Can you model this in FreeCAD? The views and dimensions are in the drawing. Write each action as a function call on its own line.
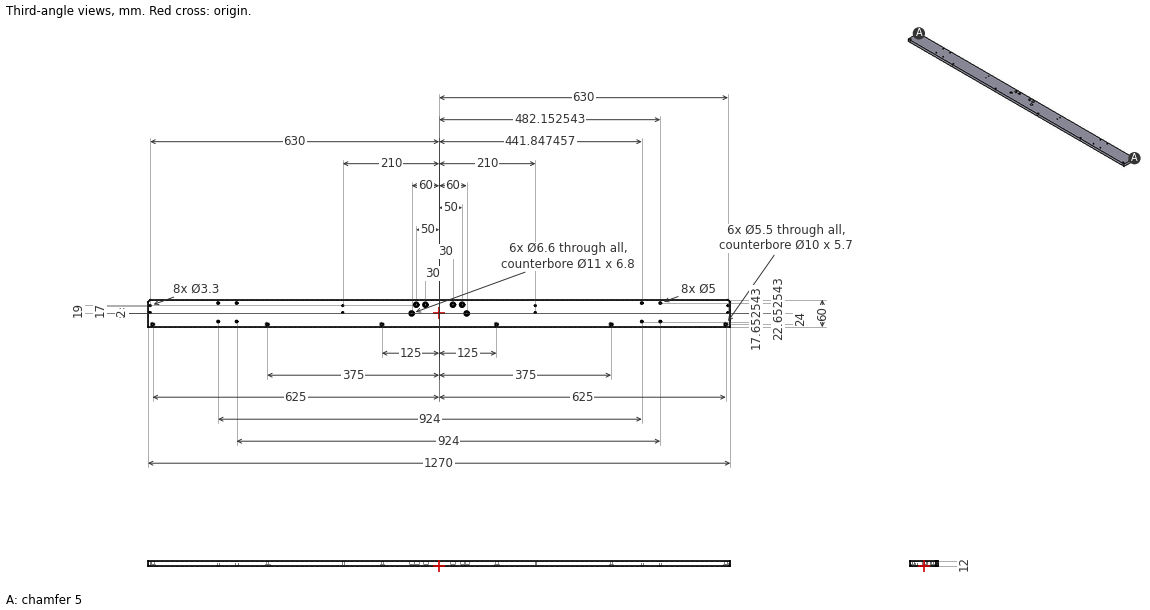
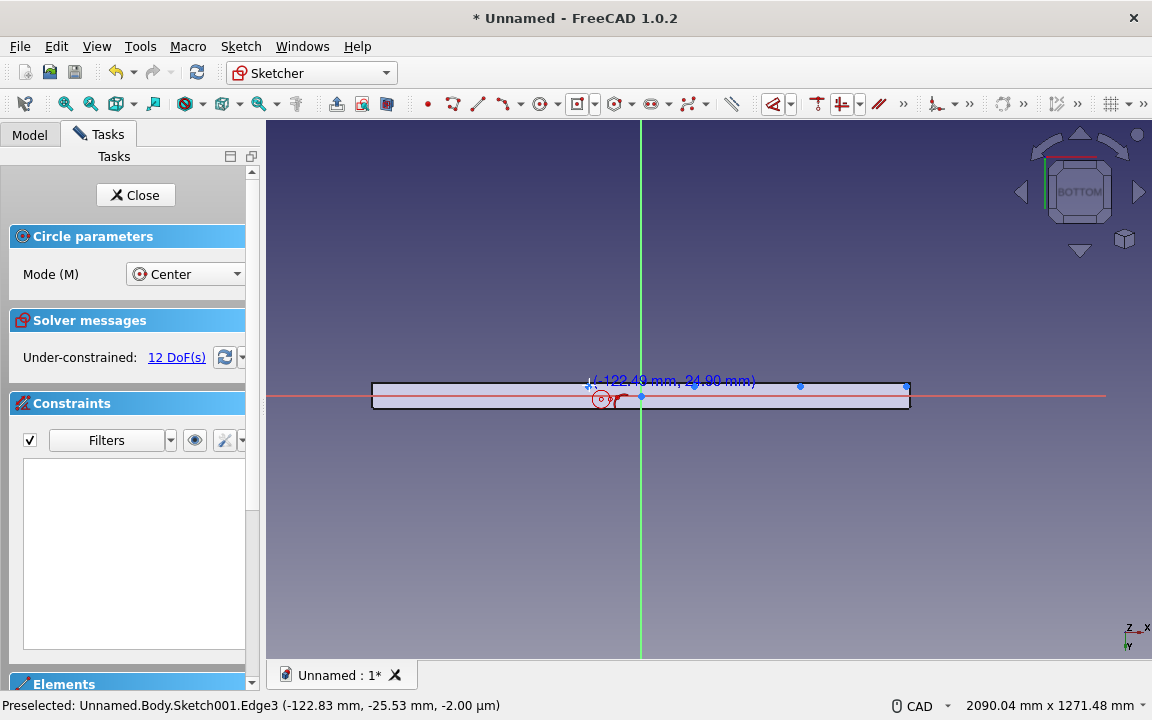
scroll(482, 386, up, 15)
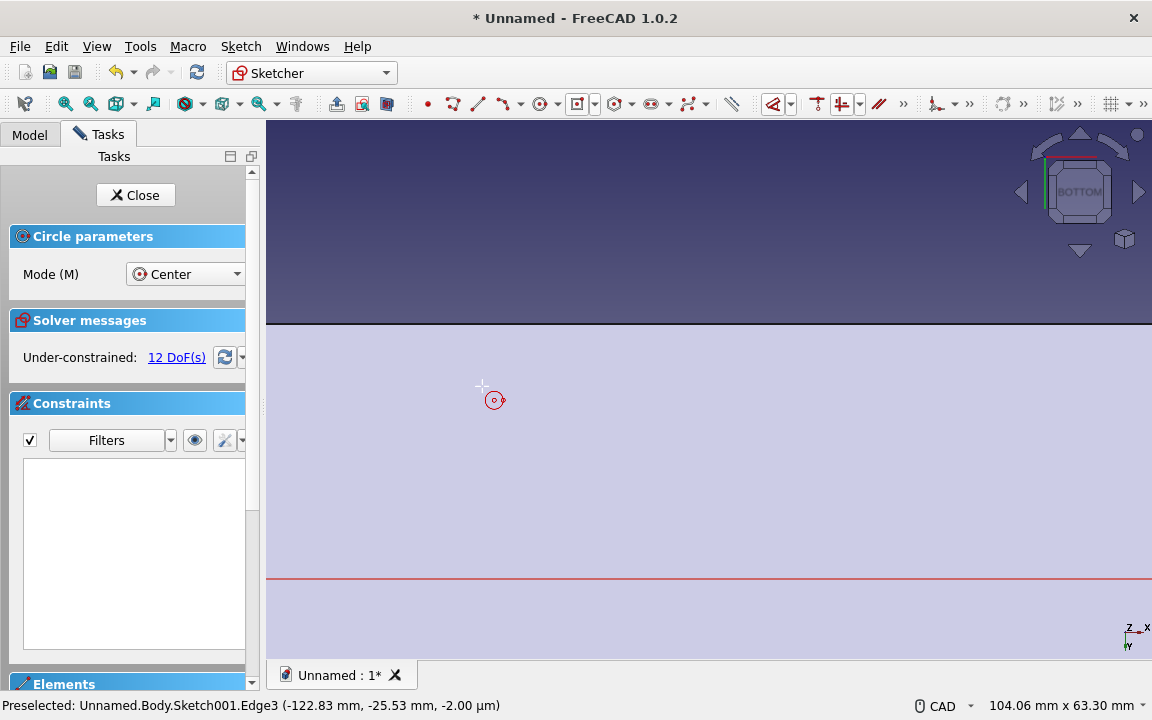
scroll(481, 386, down, 15)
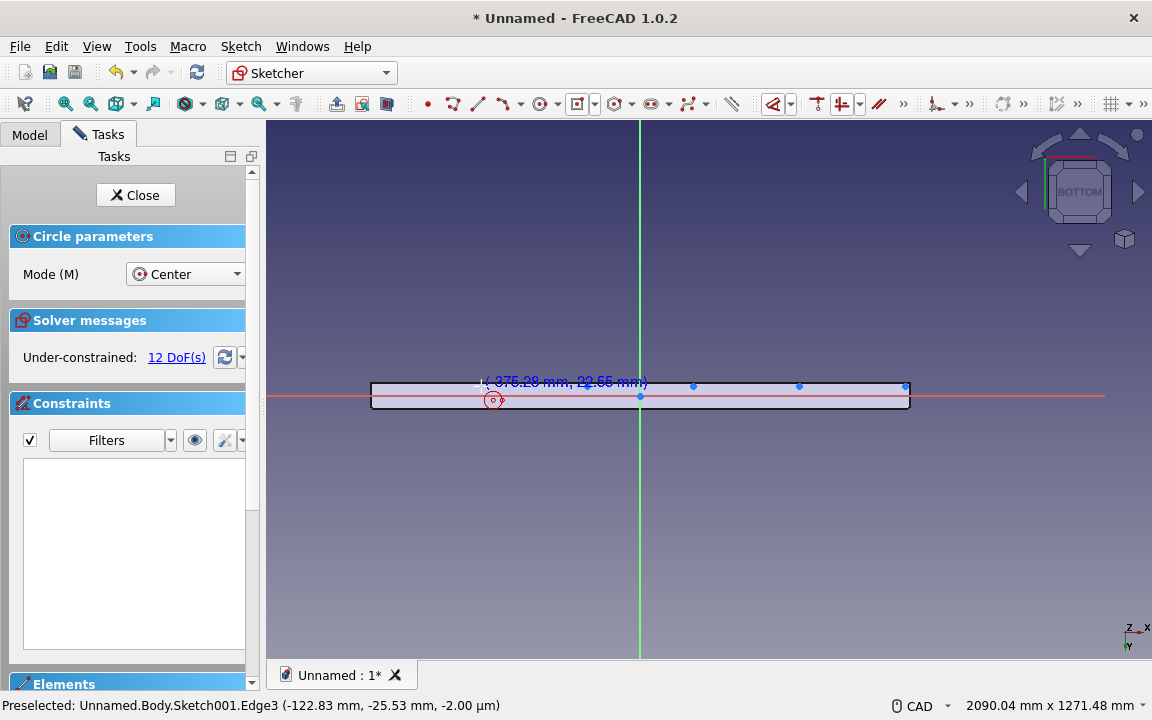
scroll(481, 386, up, 3)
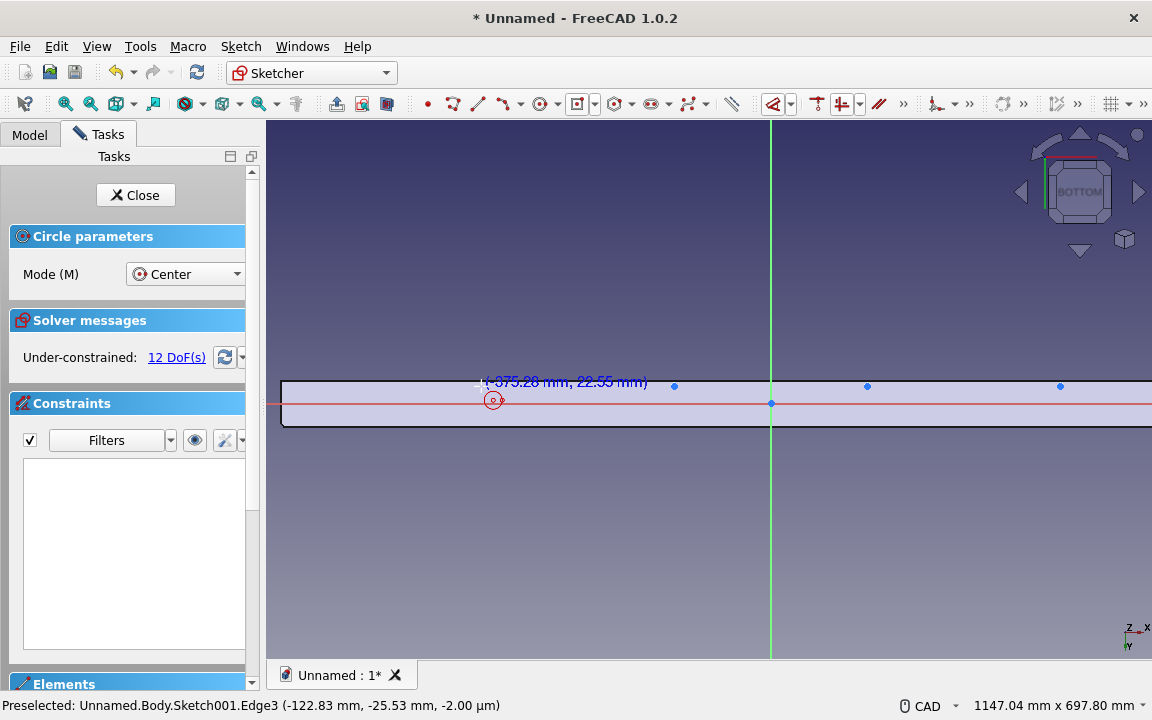
click(481, 385)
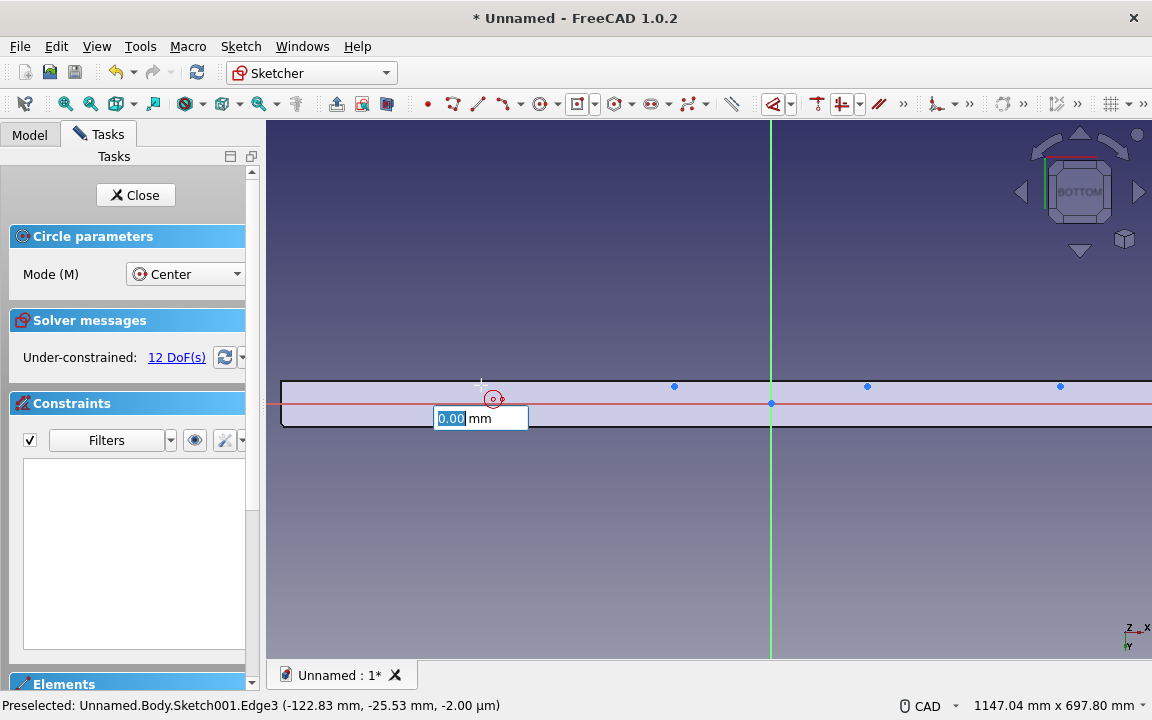
scroll(483, 384, up, 11)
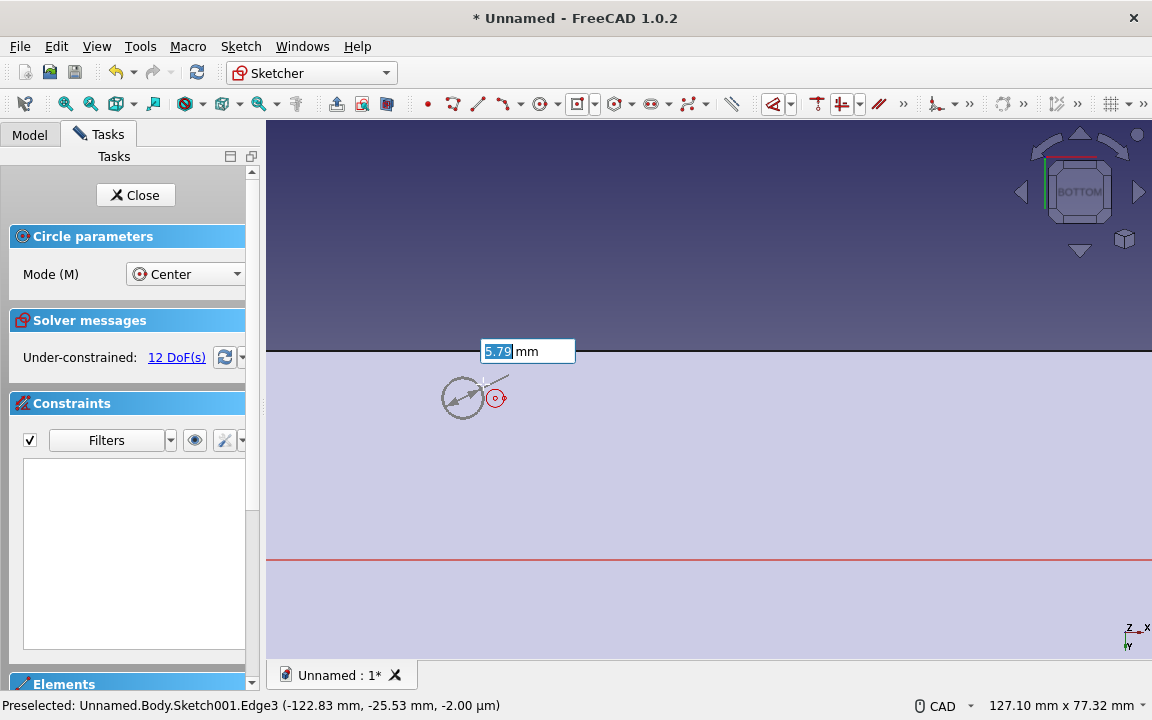
click(480, 379)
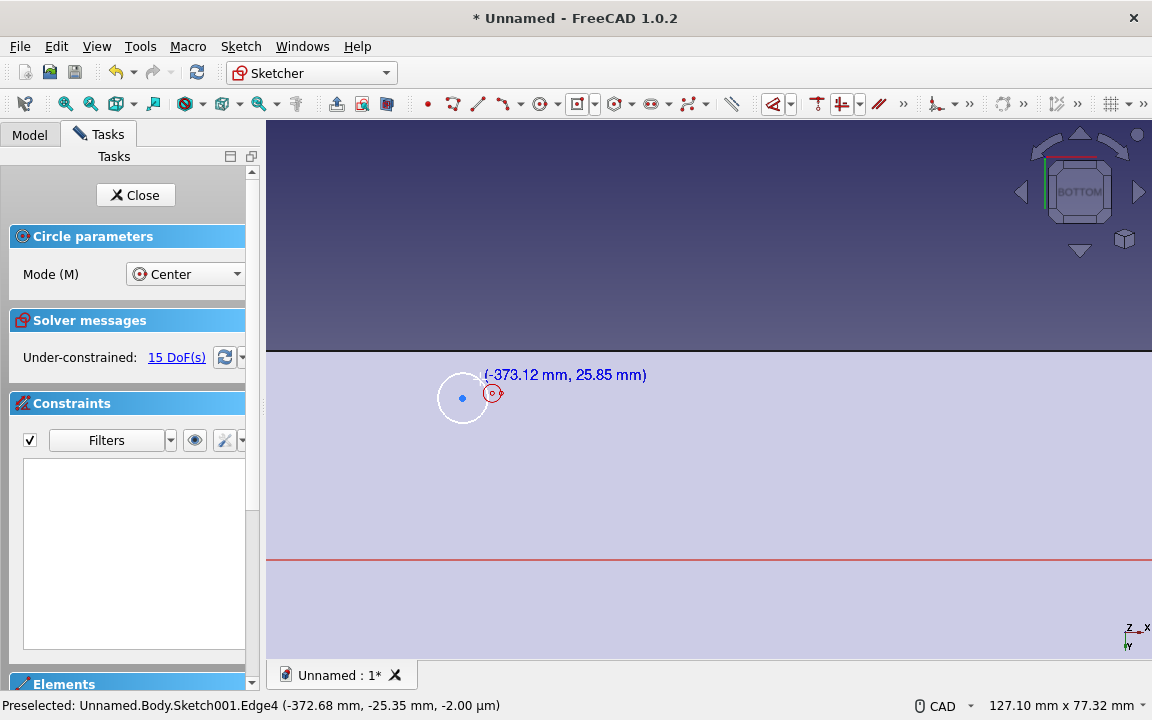
scroll(482, 384, down, 14)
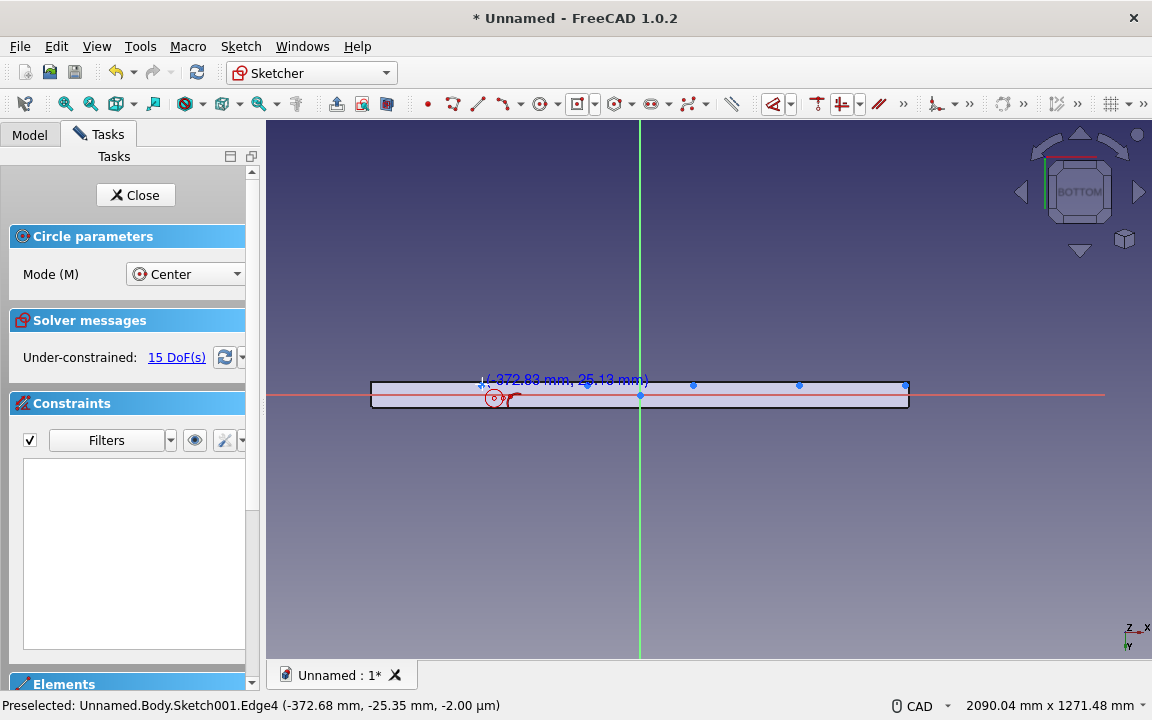
scroll(375, 385, up, 15)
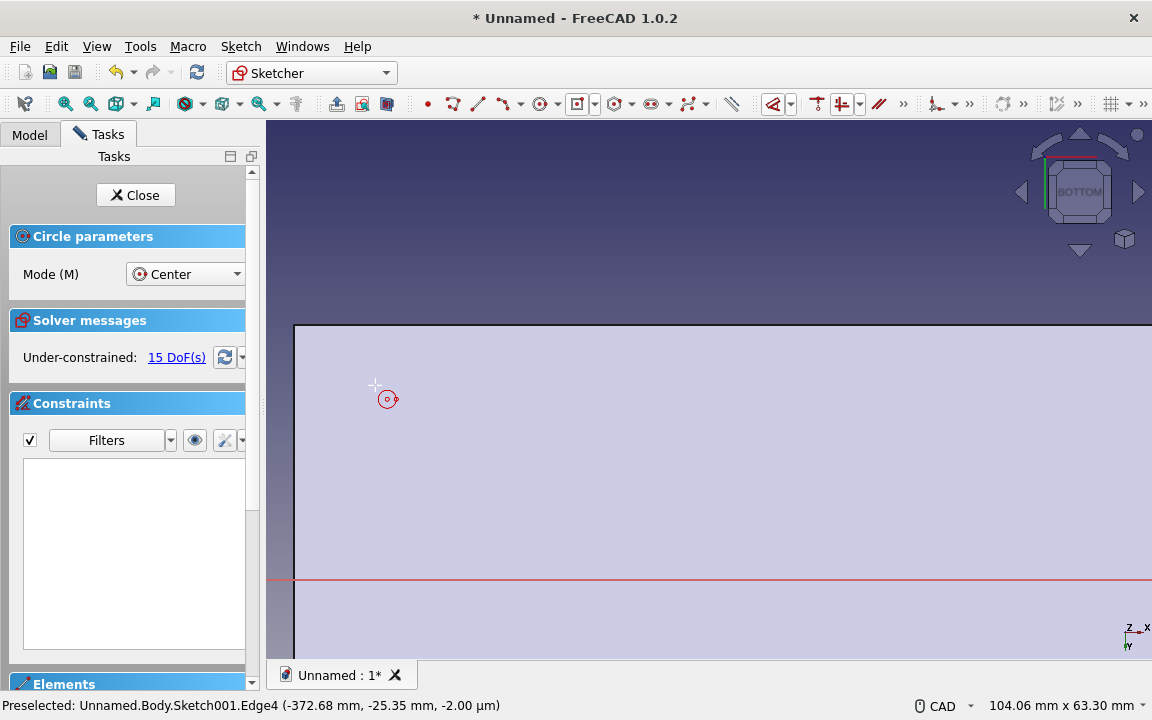
scroll(375, 385, down, 15)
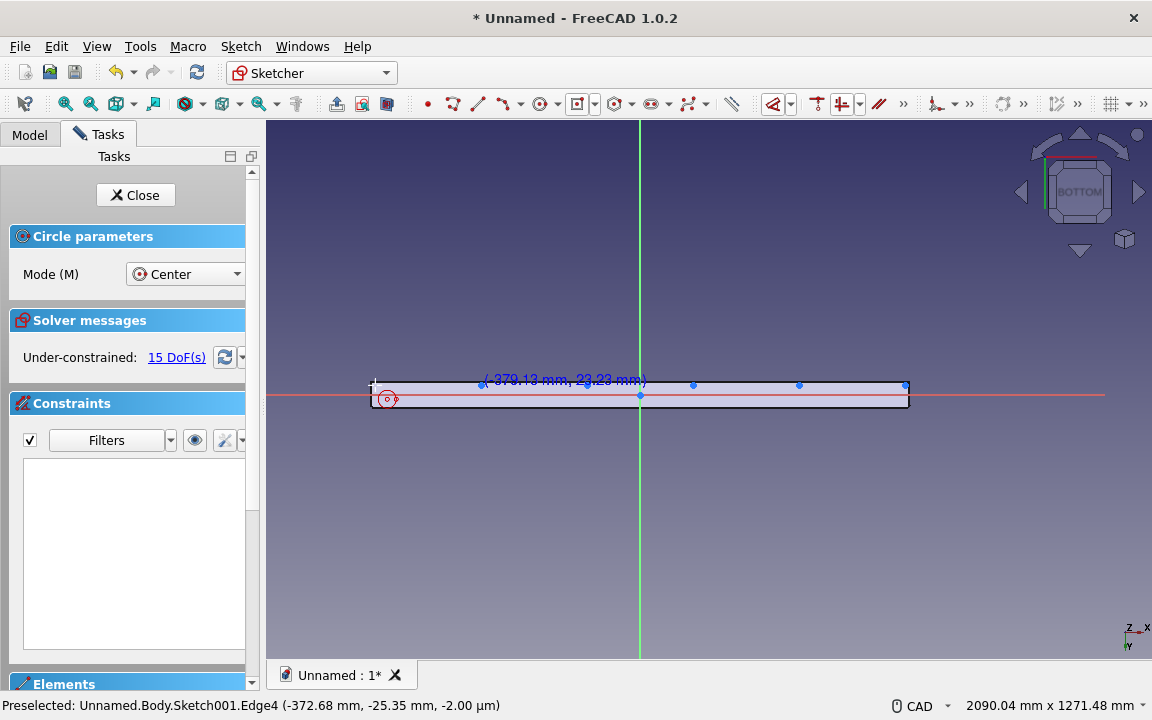
scroll(375, 385, up, 3)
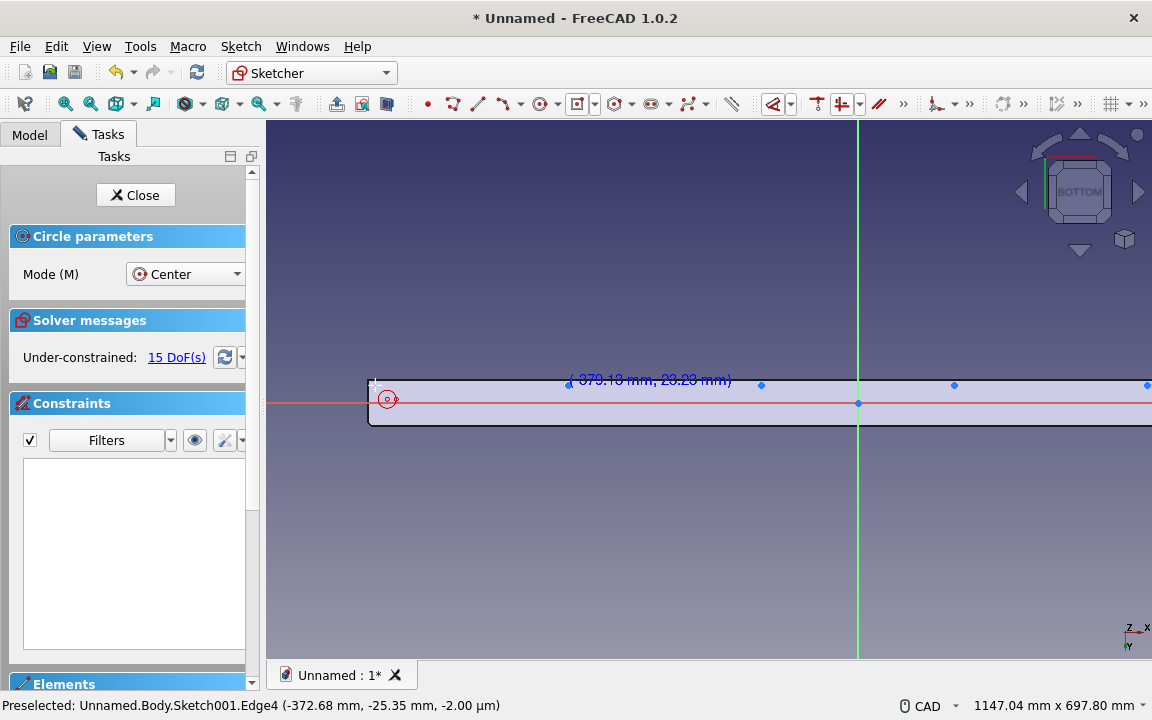
click(376, 385)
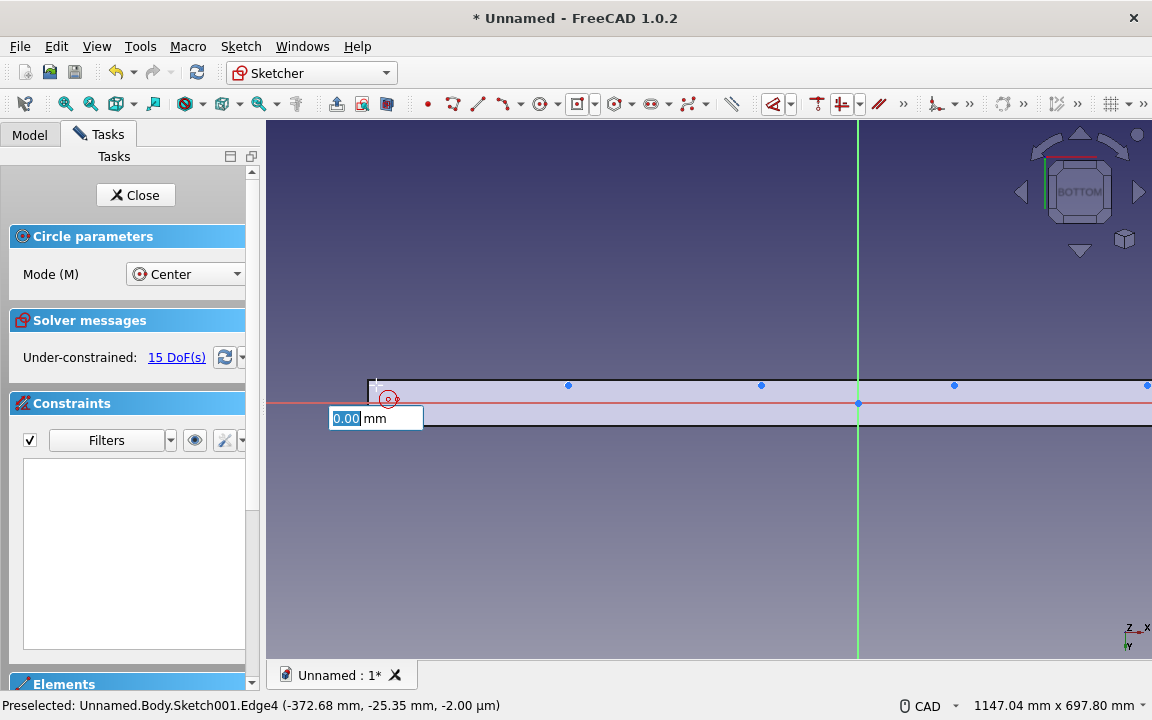
scroll(377, 383, up, 11)